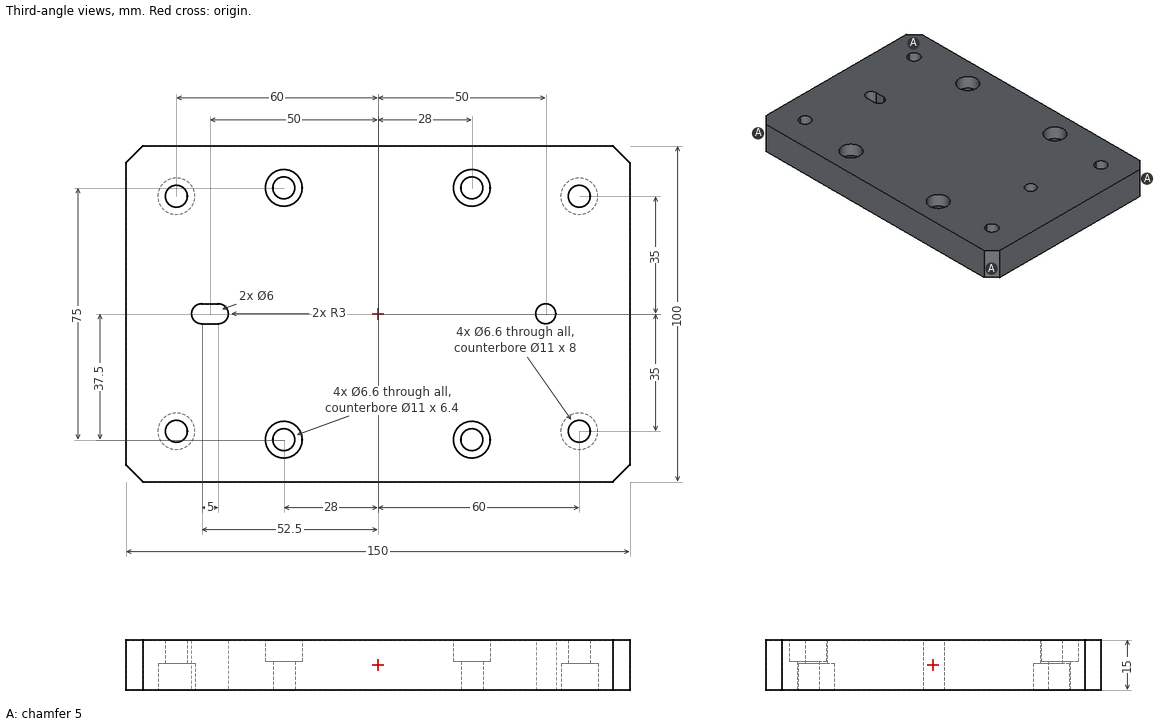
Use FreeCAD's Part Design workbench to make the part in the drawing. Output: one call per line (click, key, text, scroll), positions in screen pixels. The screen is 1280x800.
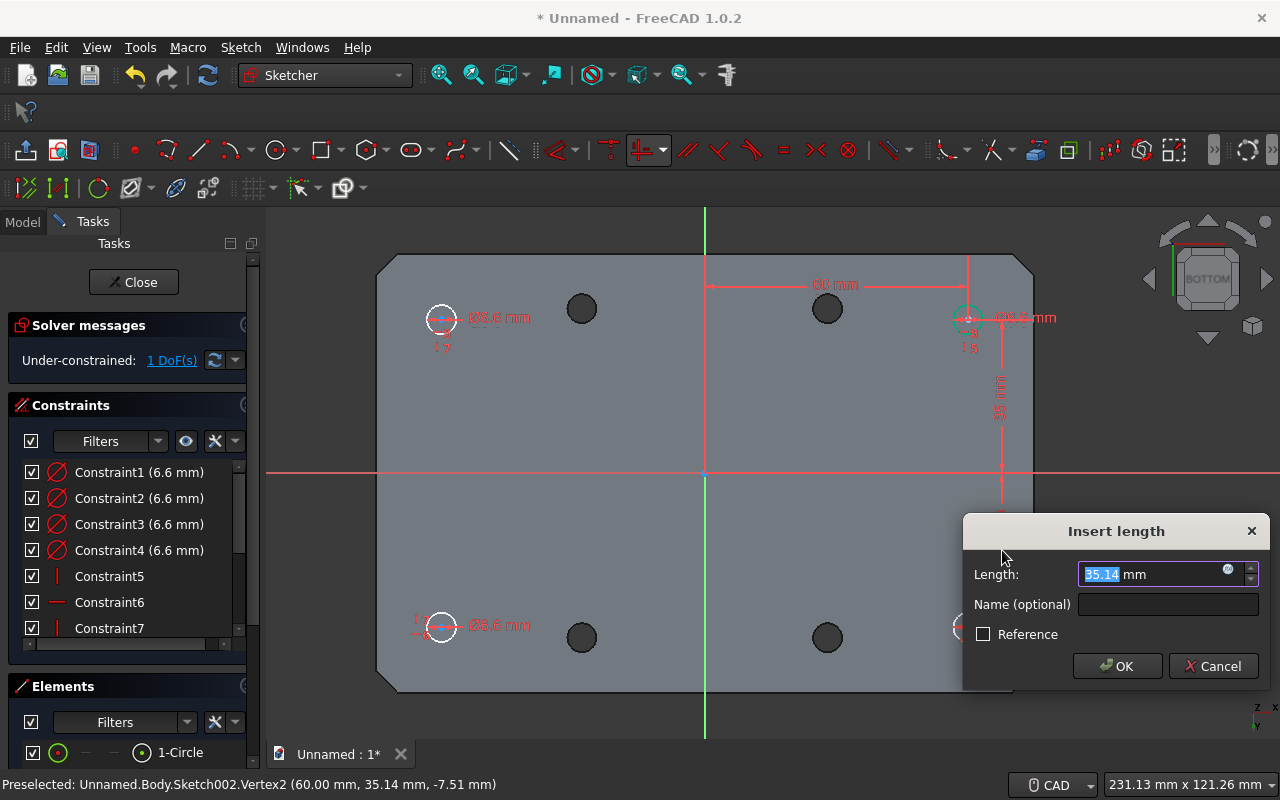
text(35)
key(Return)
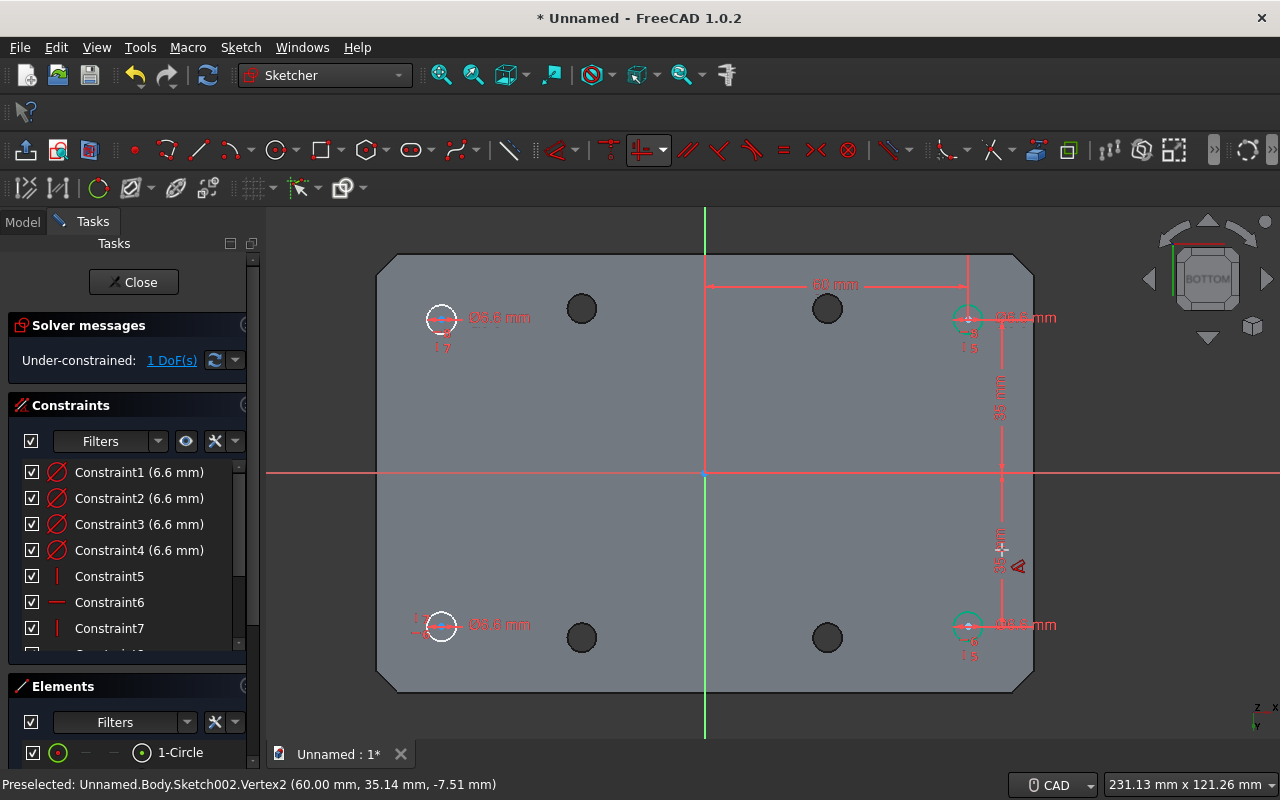
click(442, 627)
click(573, 661)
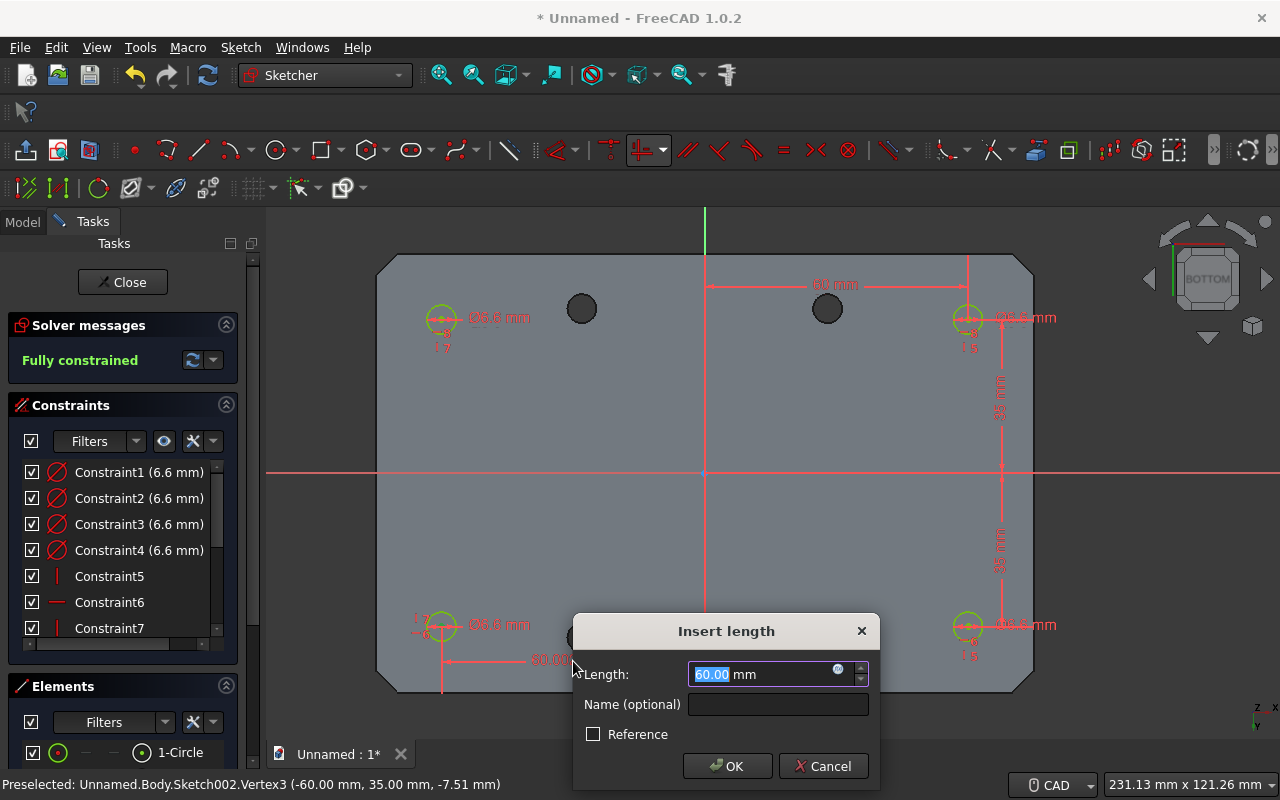
text(60)
key(Return)
key(Escape)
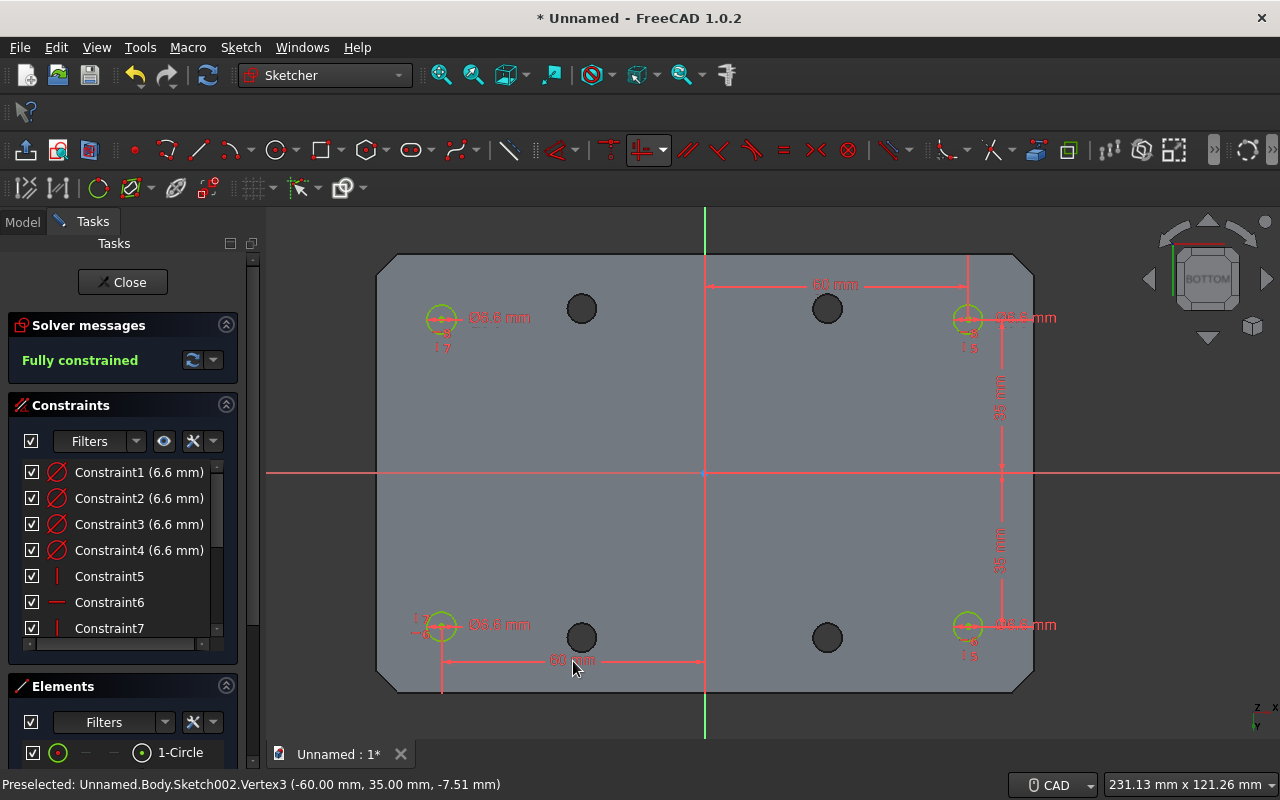
click(123, 282)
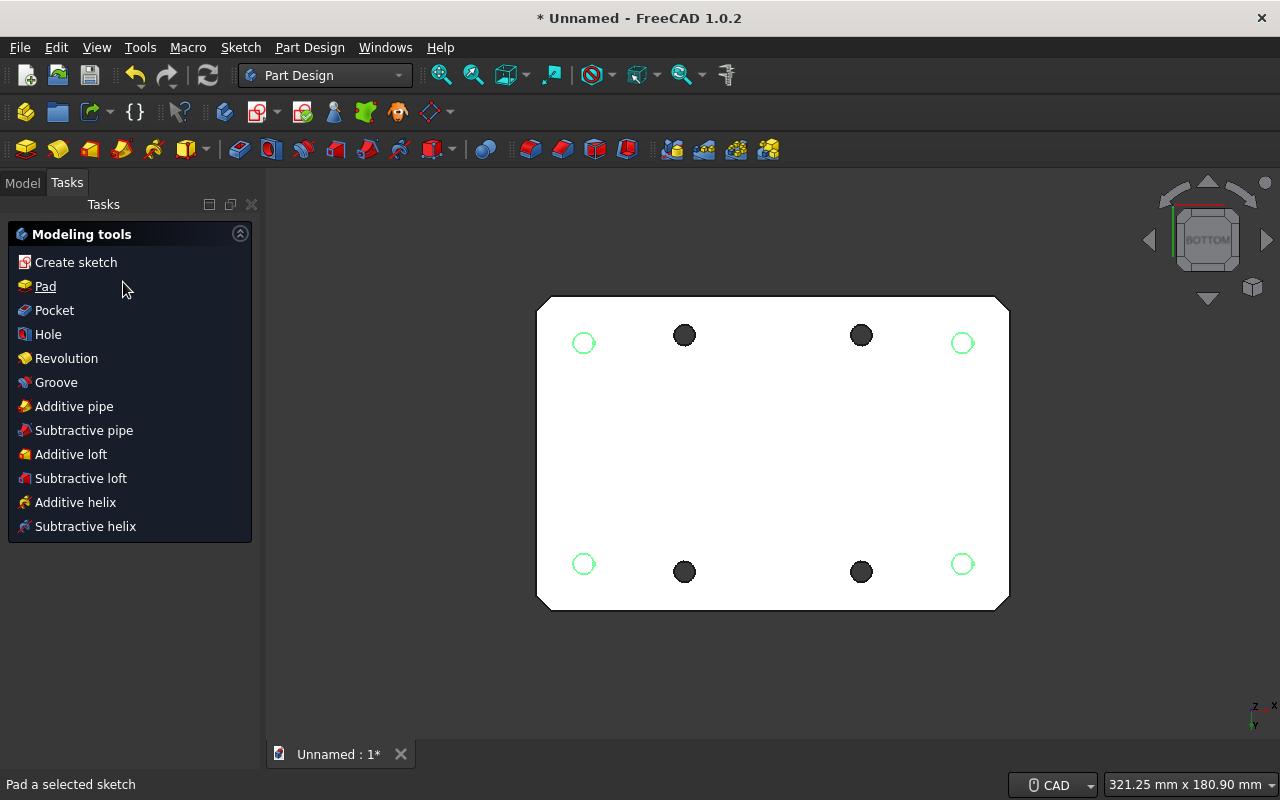
click(272, 150)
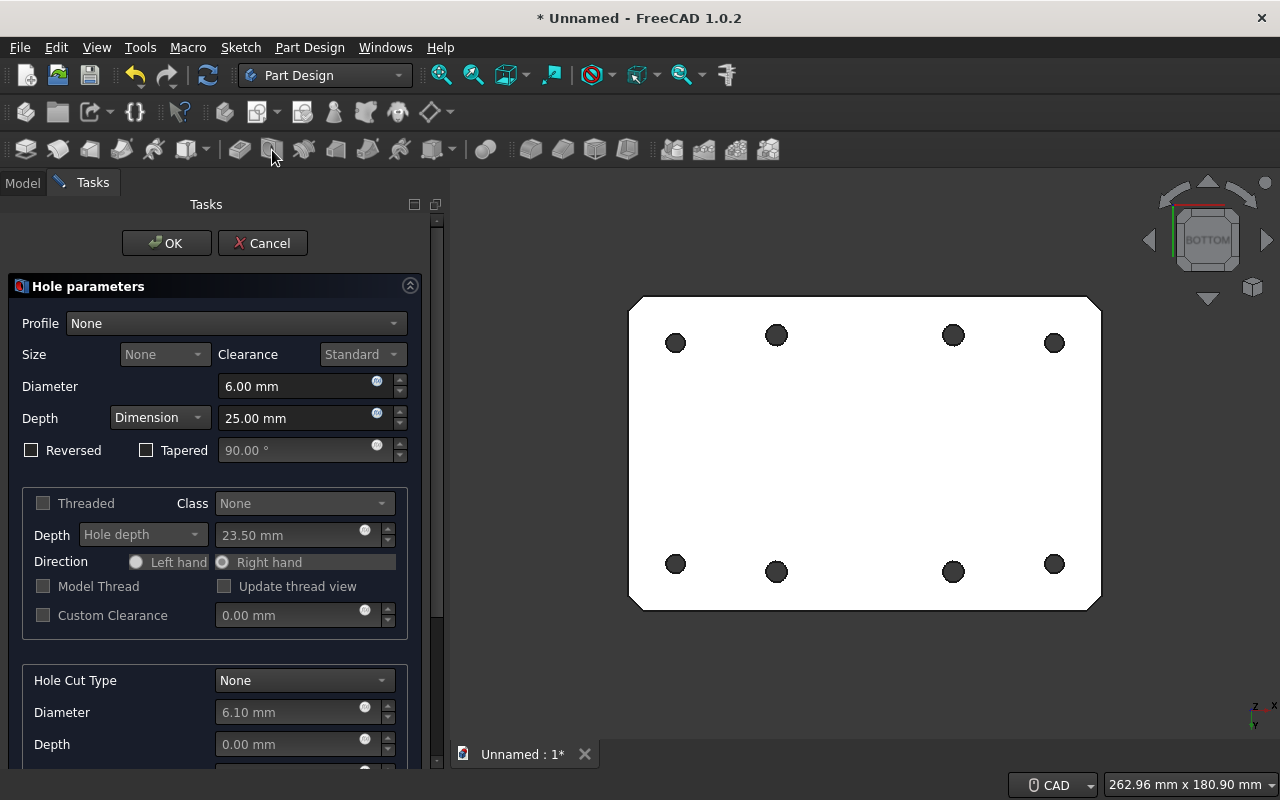
triple_click(305, 386)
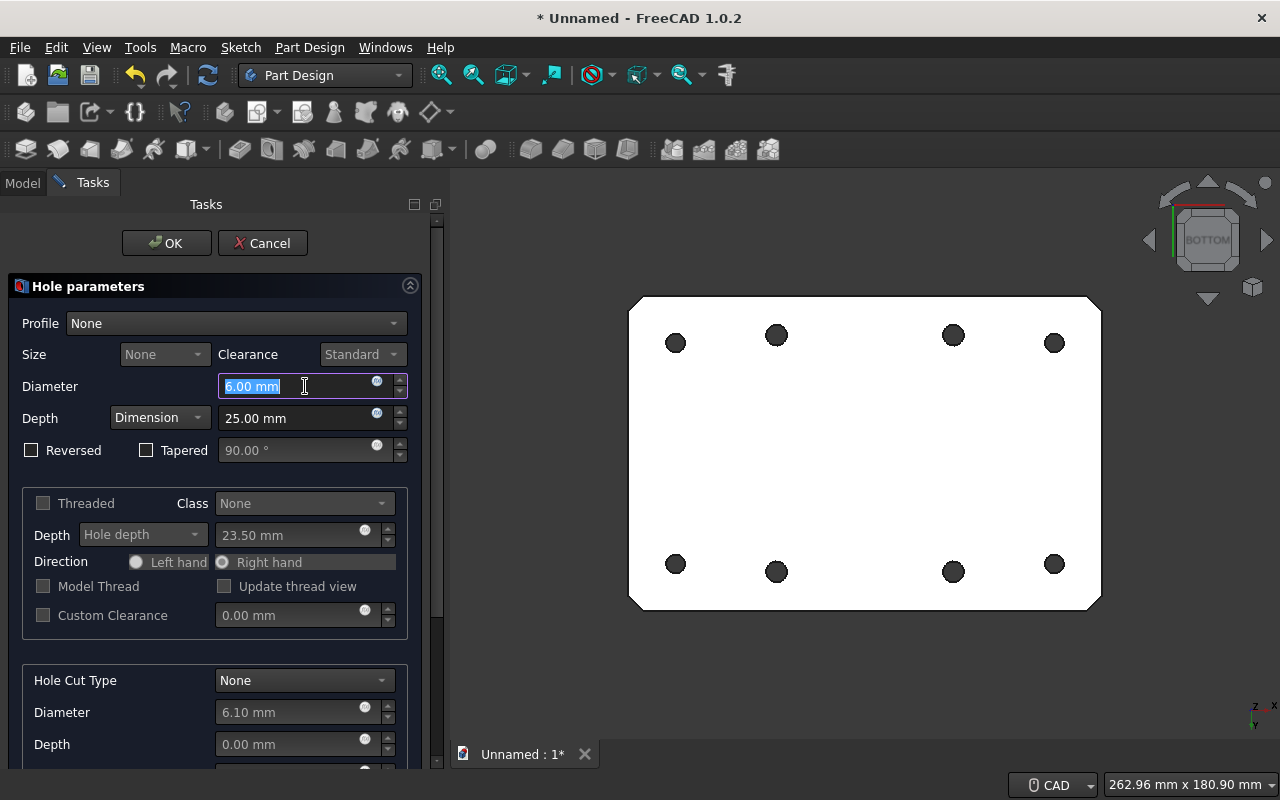
text(6.6)
key(Tab)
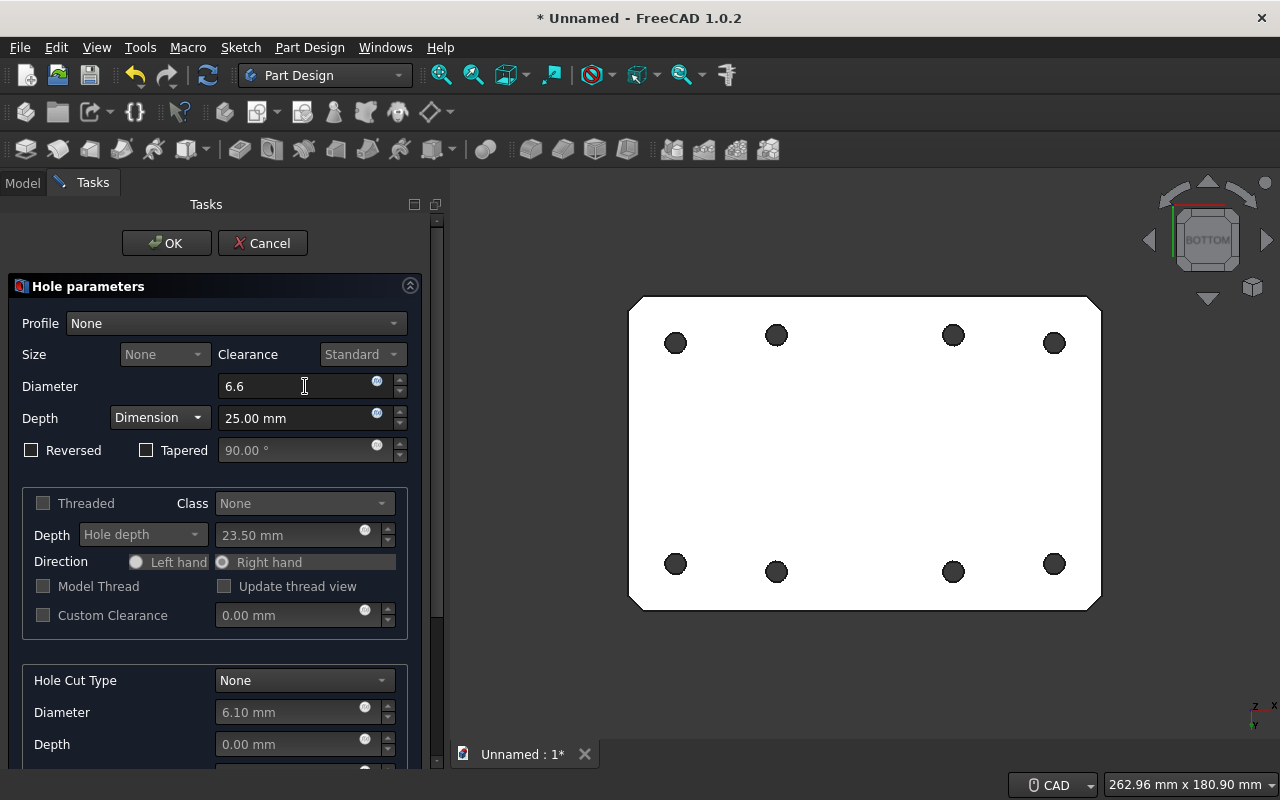
click(161, 418)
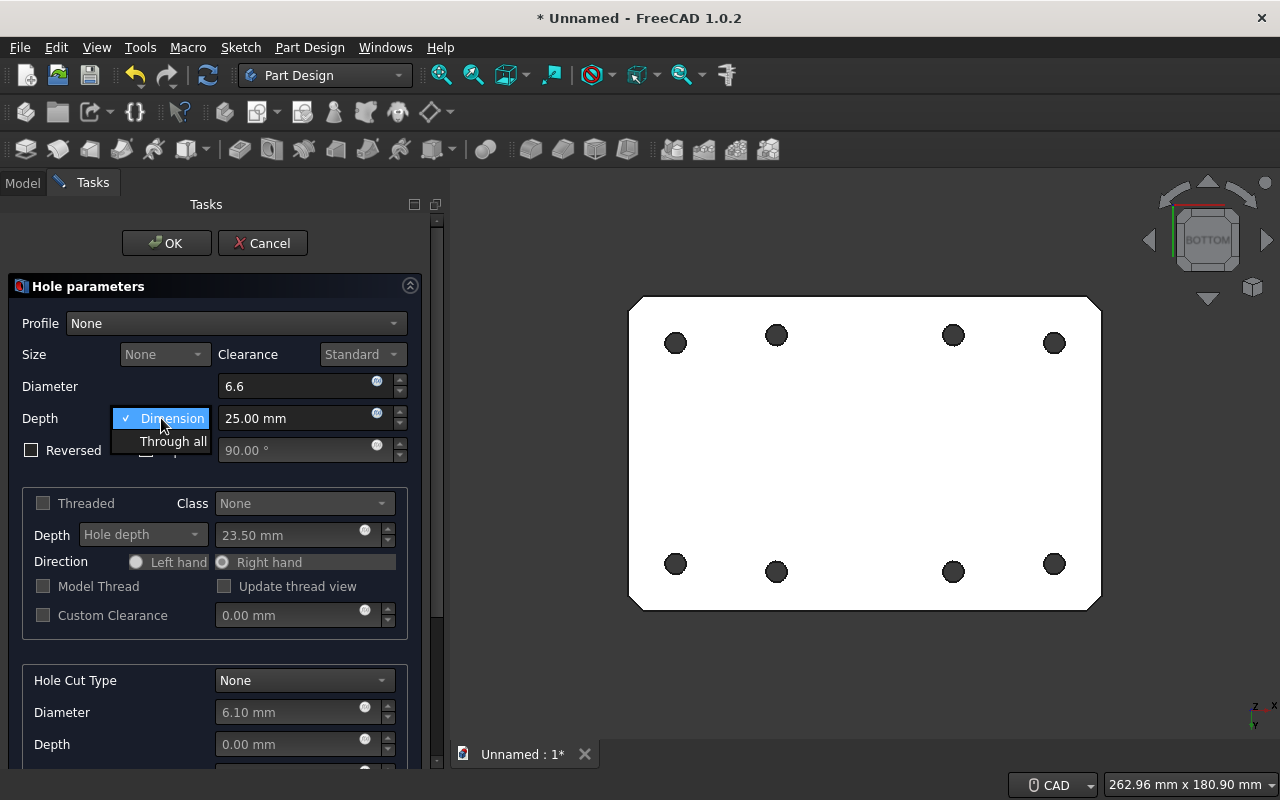
click(160, 442)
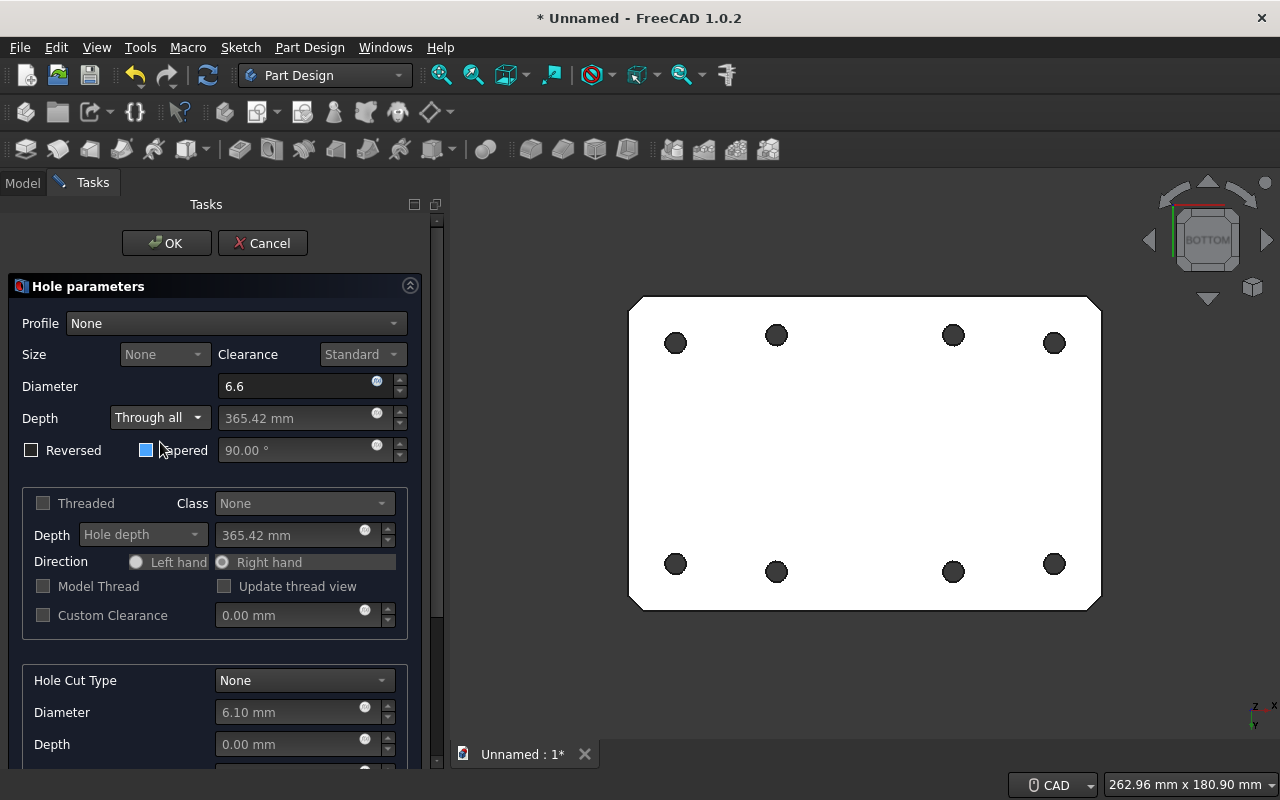
click(306, 680)